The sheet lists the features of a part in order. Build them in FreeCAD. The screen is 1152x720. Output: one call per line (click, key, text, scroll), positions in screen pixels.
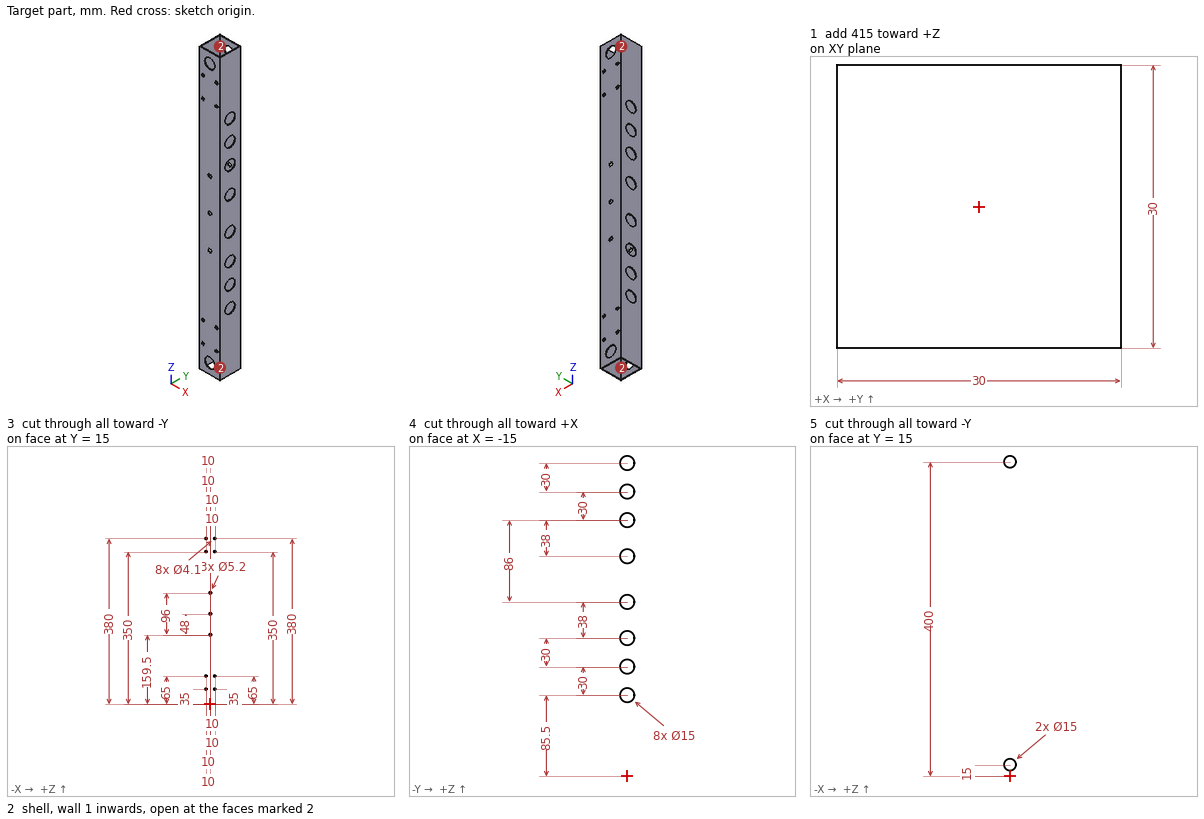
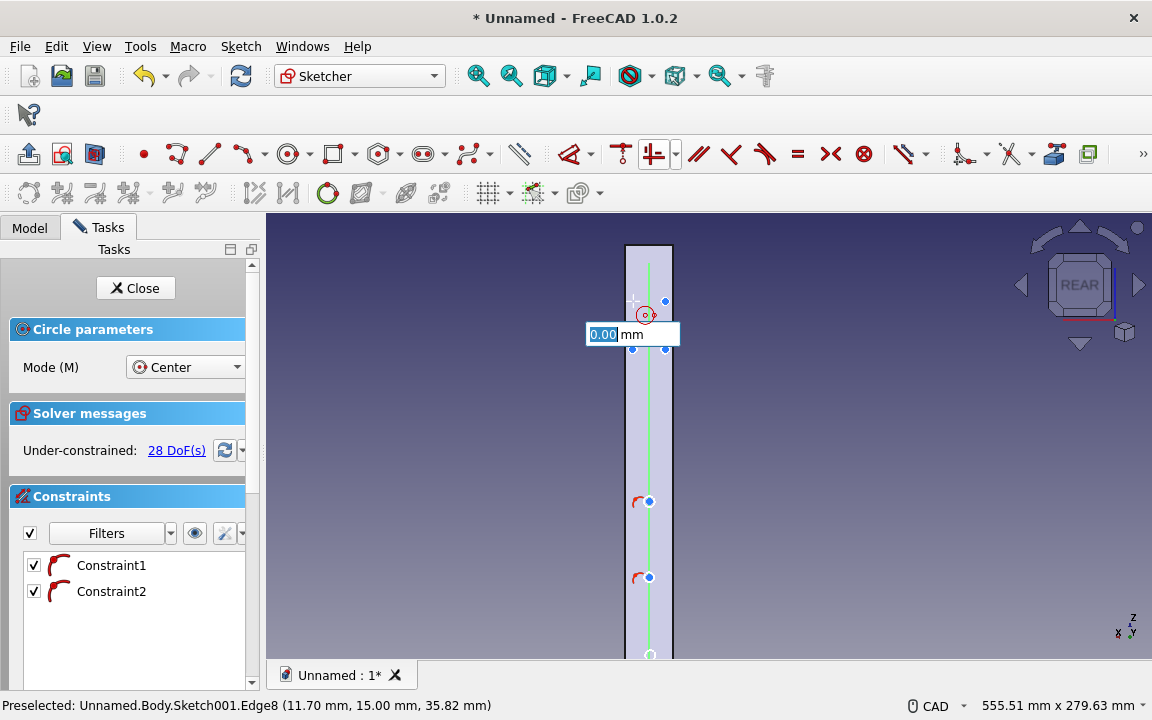
scroll(631, 298, up, 8)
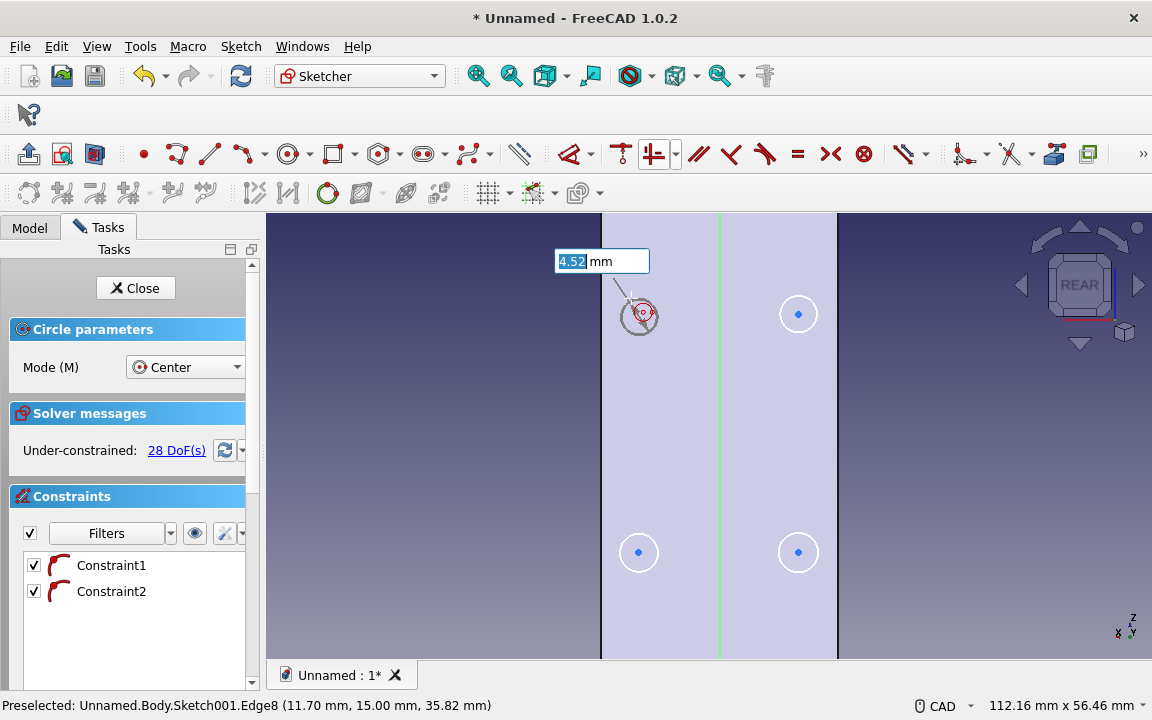
click(629, 299)
key(Escape)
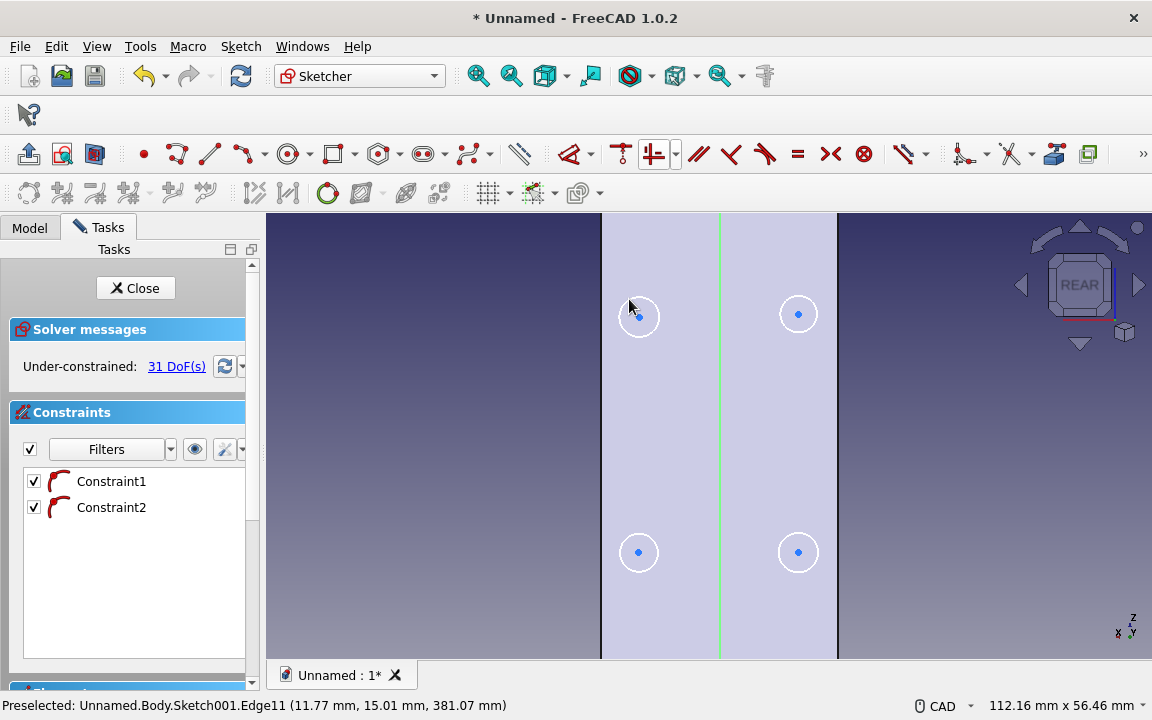
scroll(633, 300, down, 12)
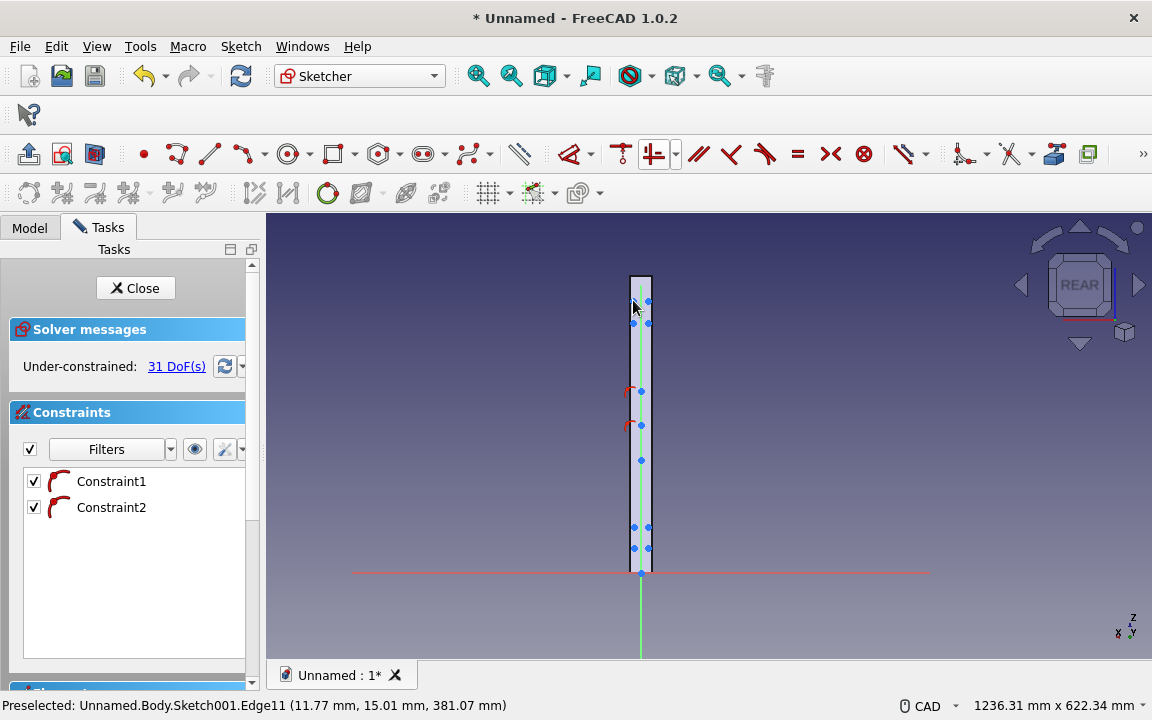
scroll(643, 459, up, 10)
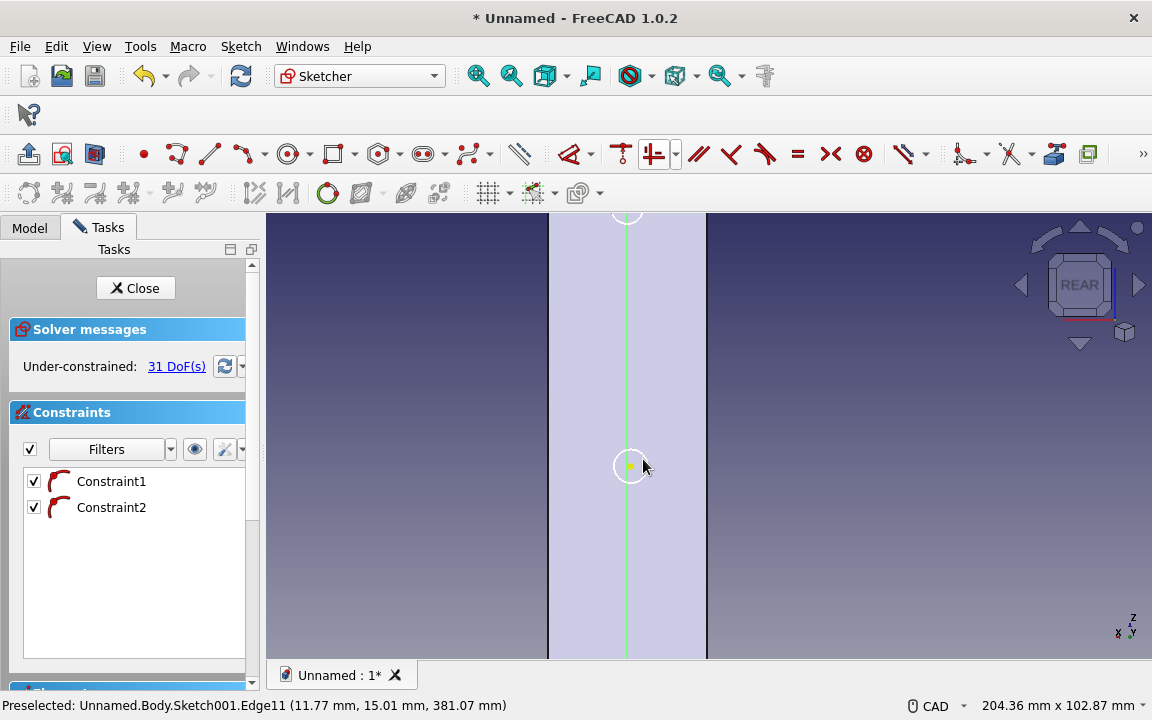
click(643, 454)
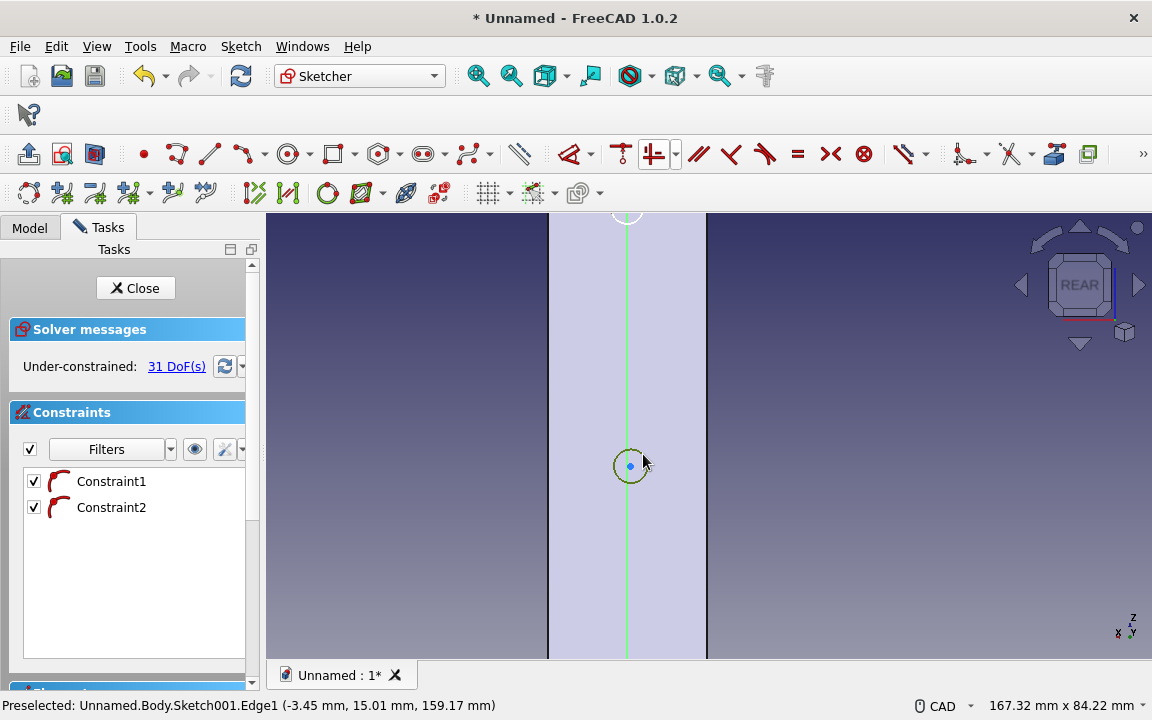
scroll(643, 459, down, 10)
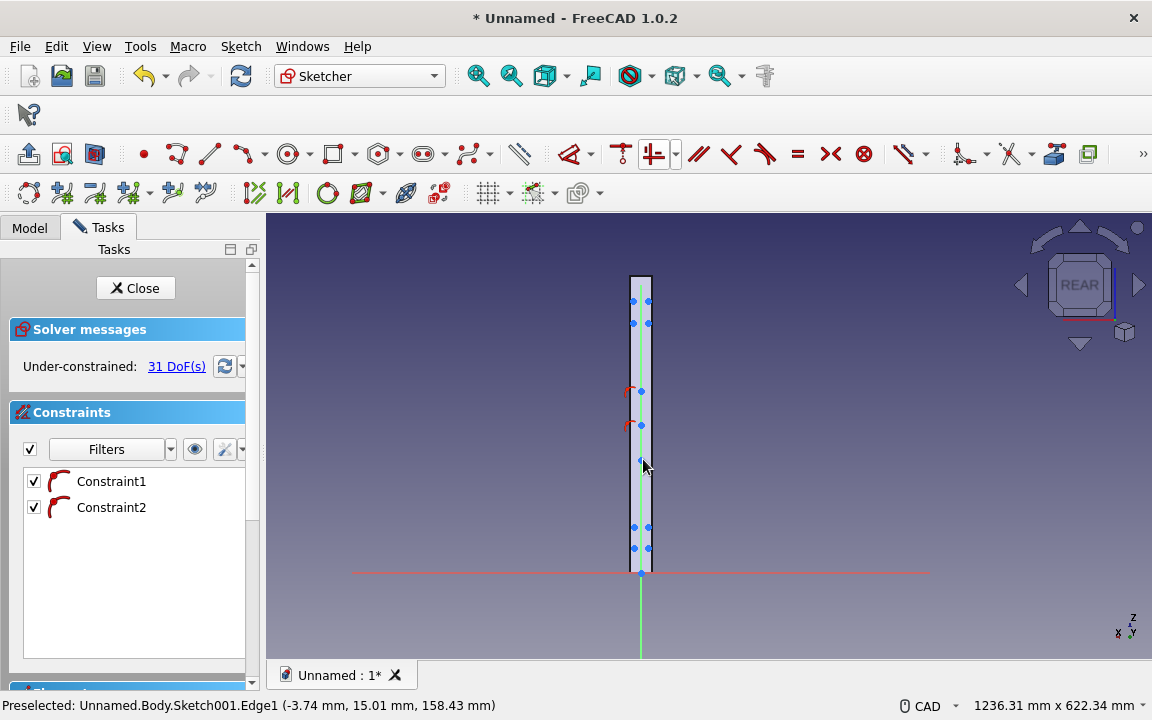
scroll(643, 390, up, 11)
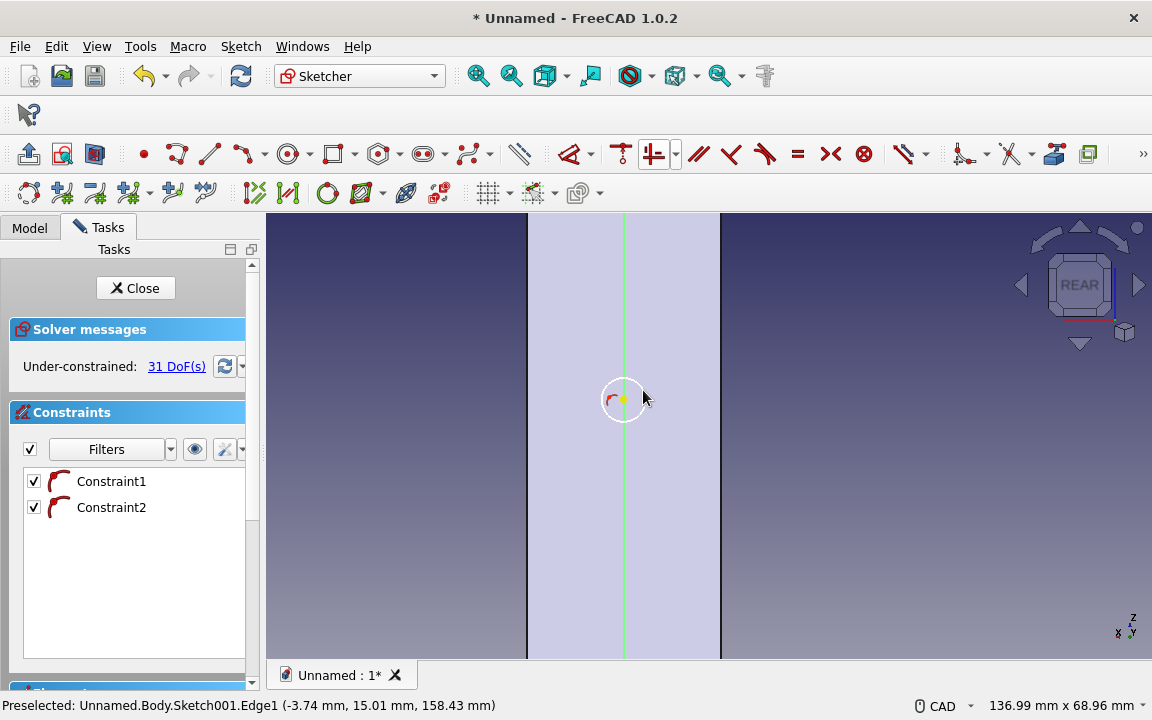
click(639, 384)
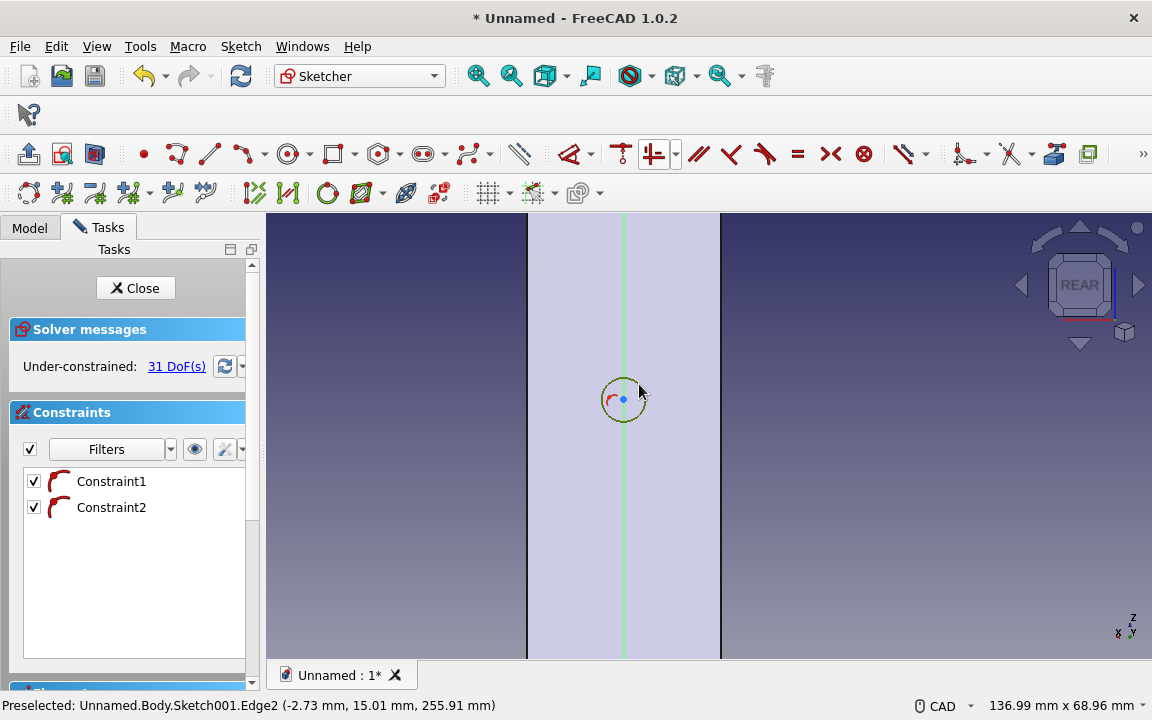
scroll(643, 390, down, 11)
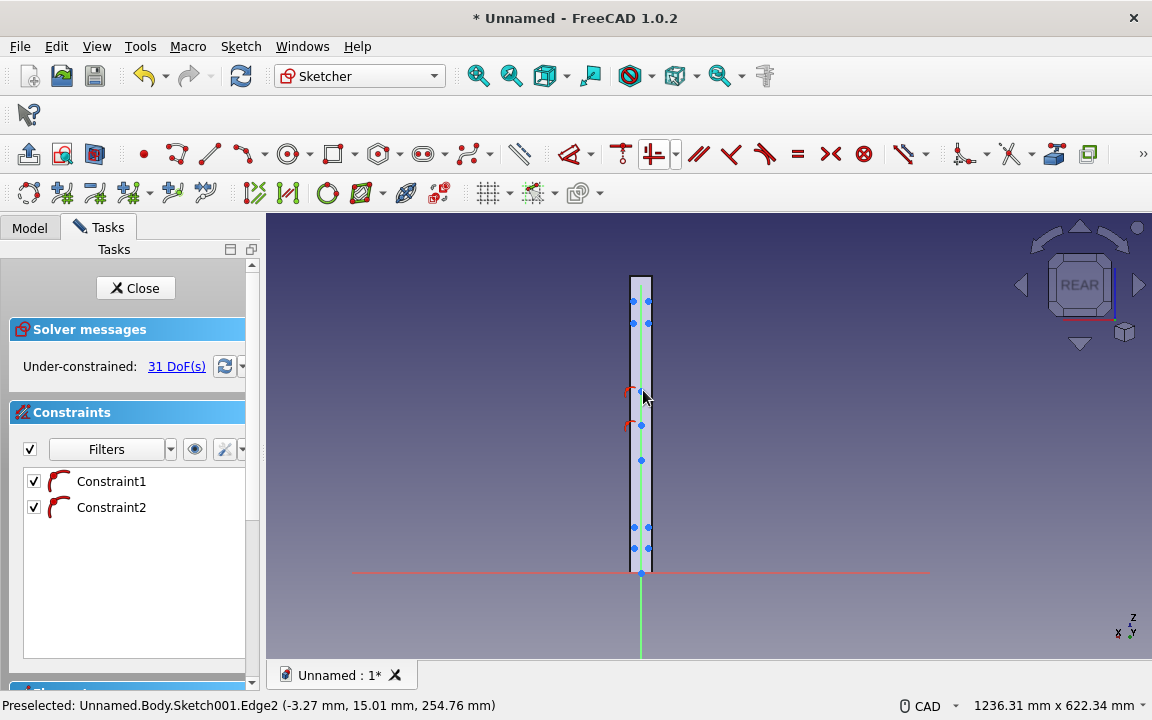
scroll(643, 424, up, 11)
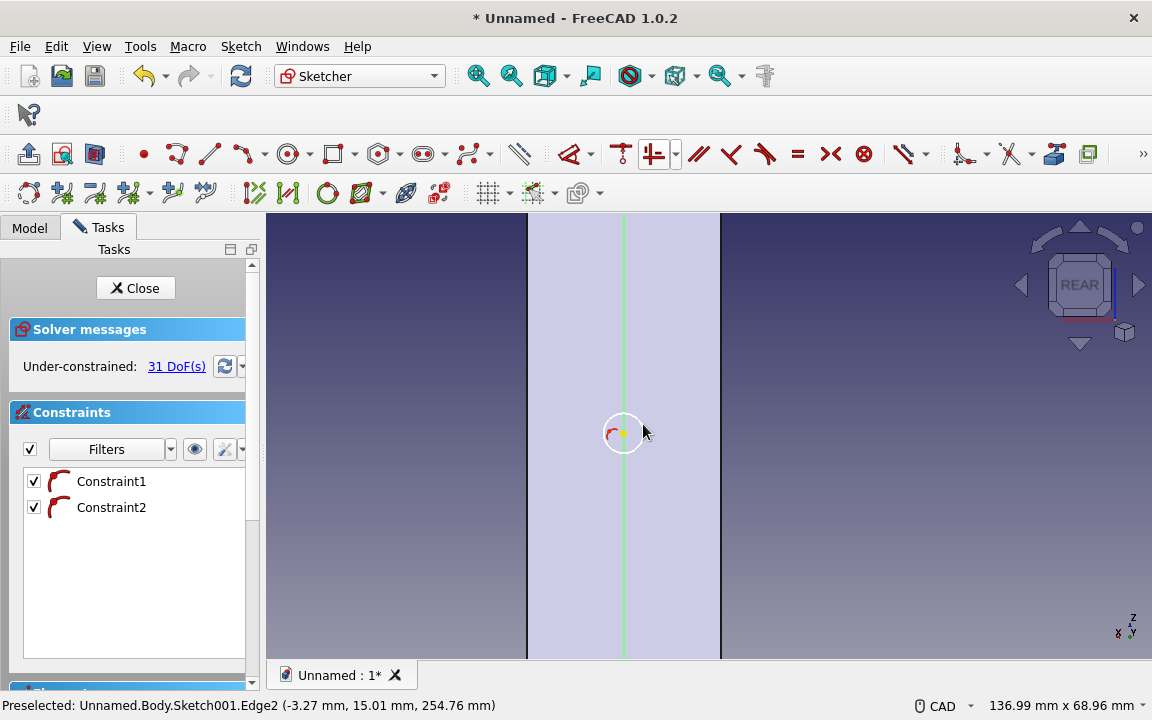
click(638, 419)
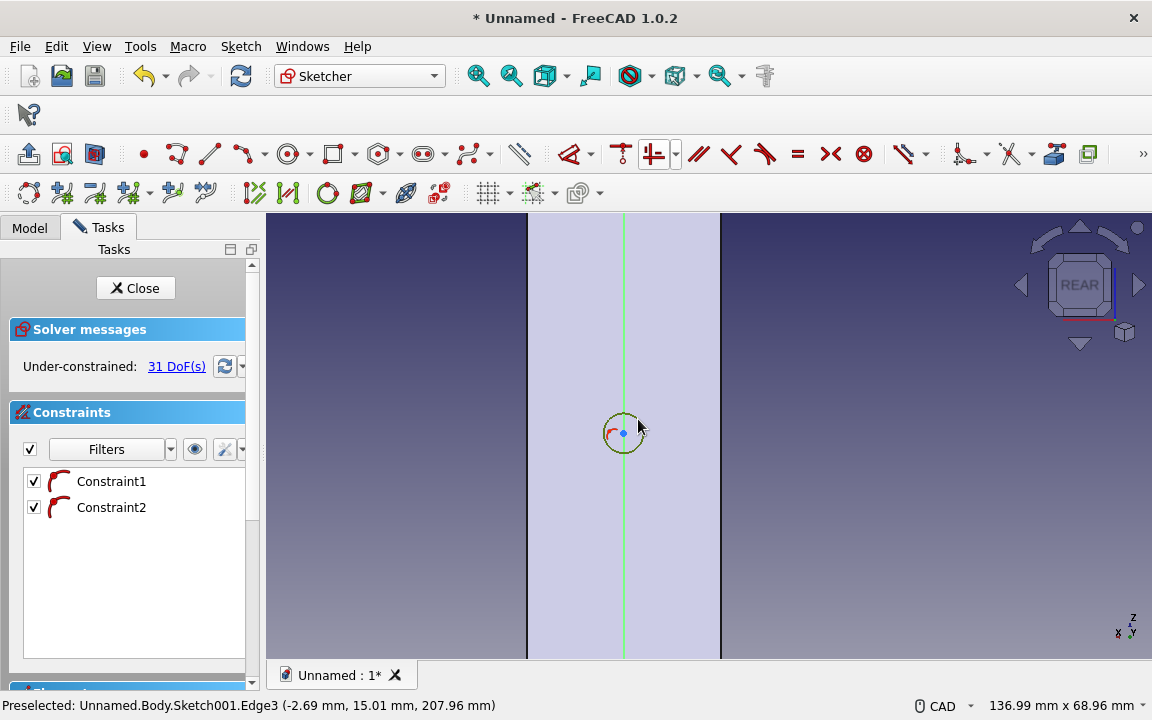
key(e)